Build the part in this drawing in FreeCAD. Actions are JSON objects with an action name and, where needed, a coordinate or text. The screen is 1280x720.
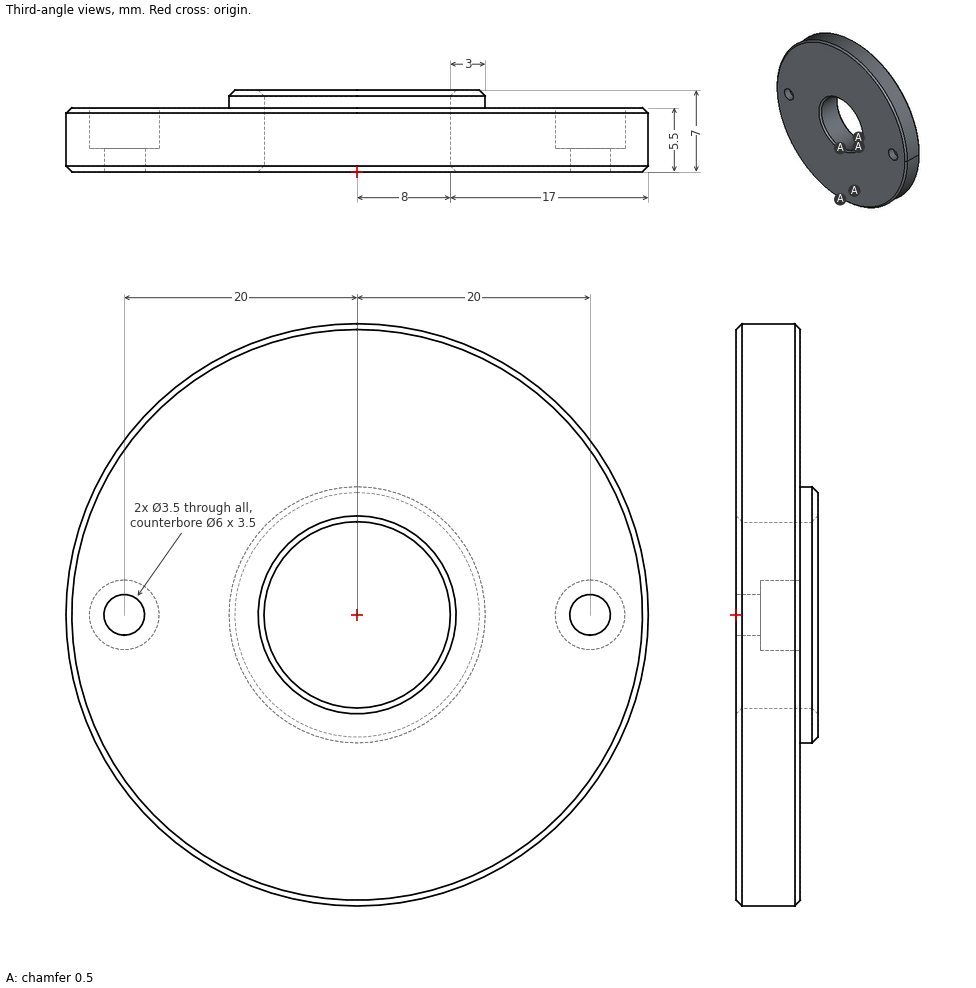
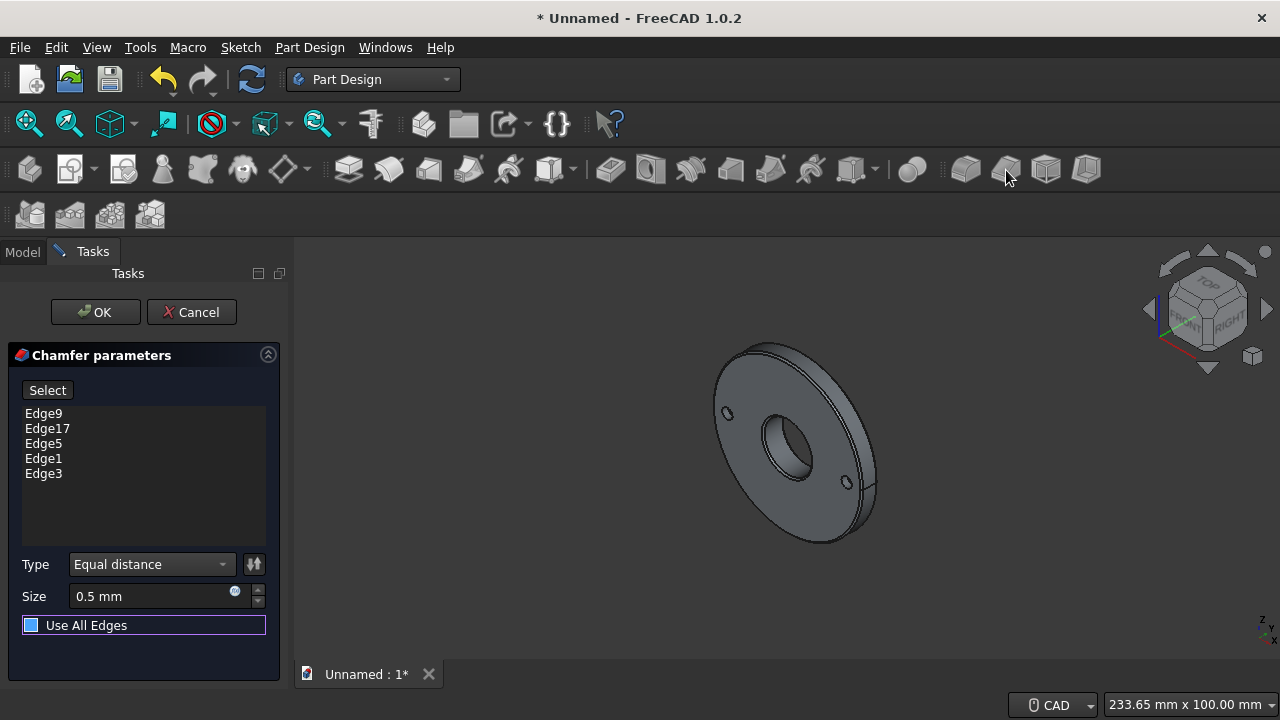
{"action": "left_click", "coordinate": [96, 312]}